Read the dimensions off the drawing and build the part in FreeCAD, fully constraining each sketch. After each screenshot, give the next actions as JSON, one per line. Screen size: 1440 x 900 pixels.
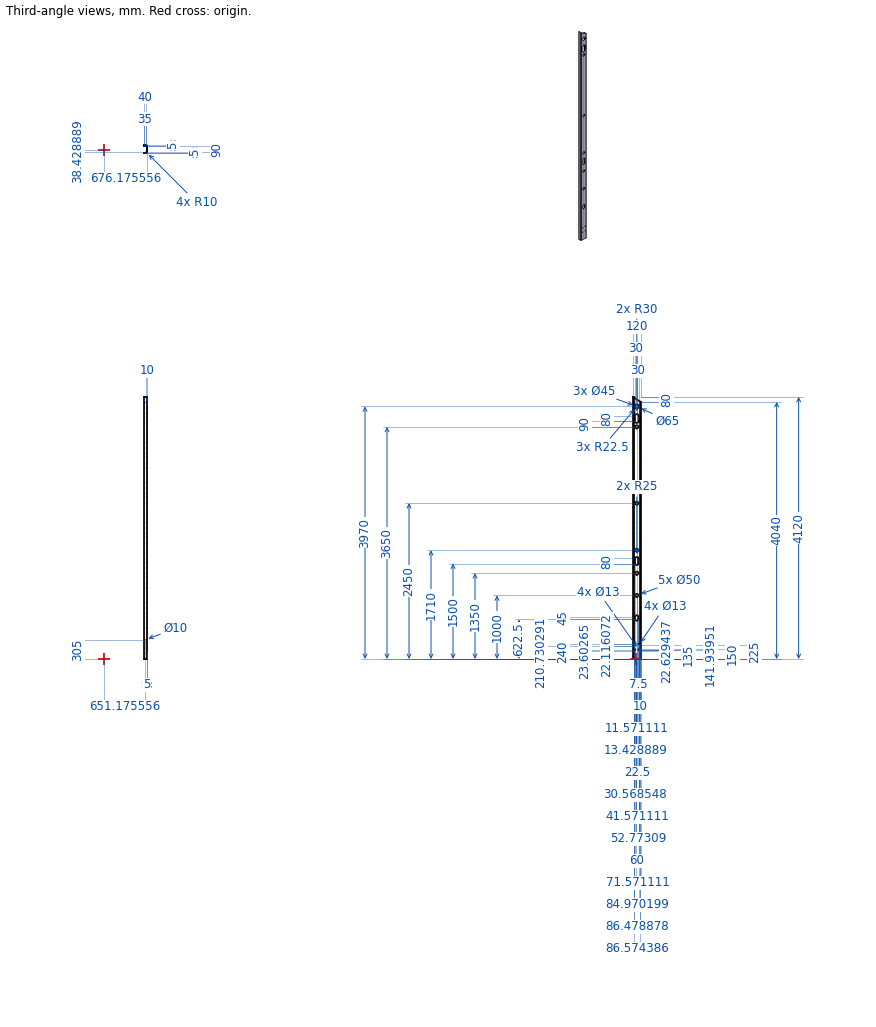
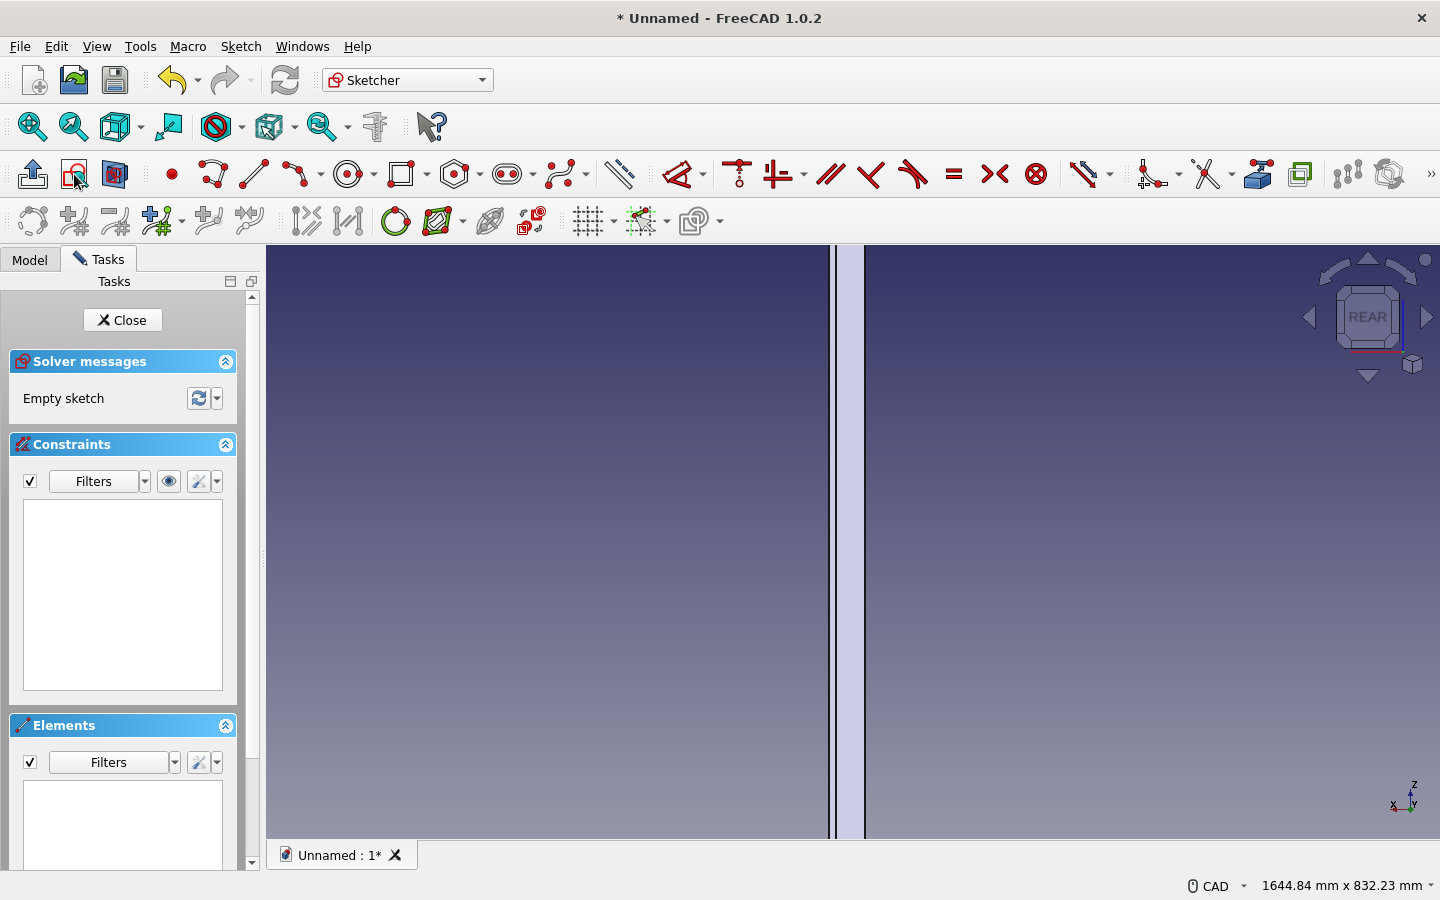
{"action": "scroll", "coordinate": [784, 542], "scroll_direction": "down", "scroll_amount": 5}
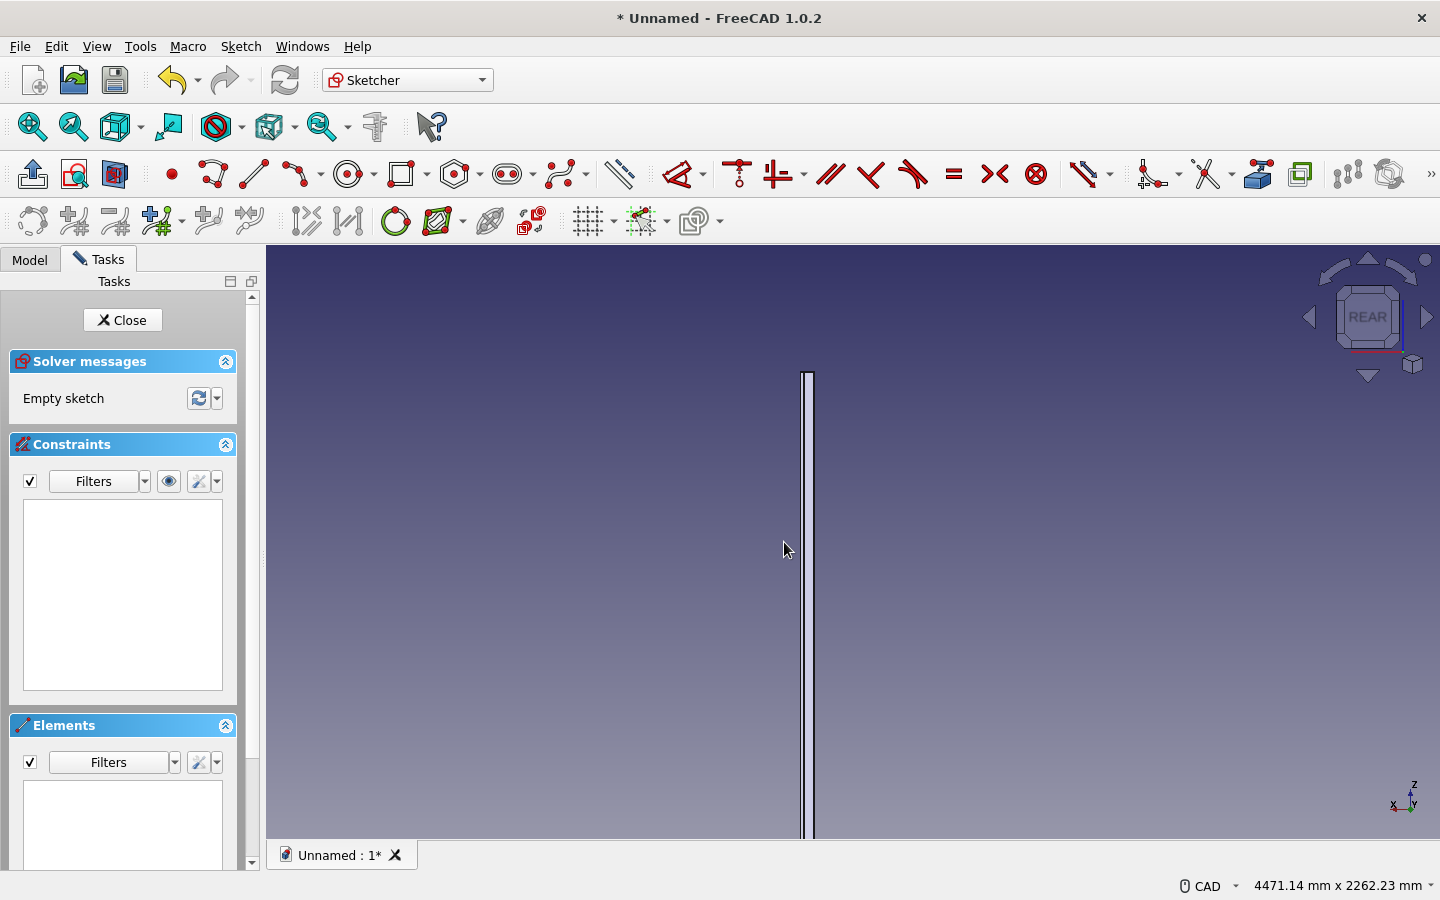
{"action": "scroll", "coordinate": [784, 542], "scroll_direction": "down", "scroll_amount": 5}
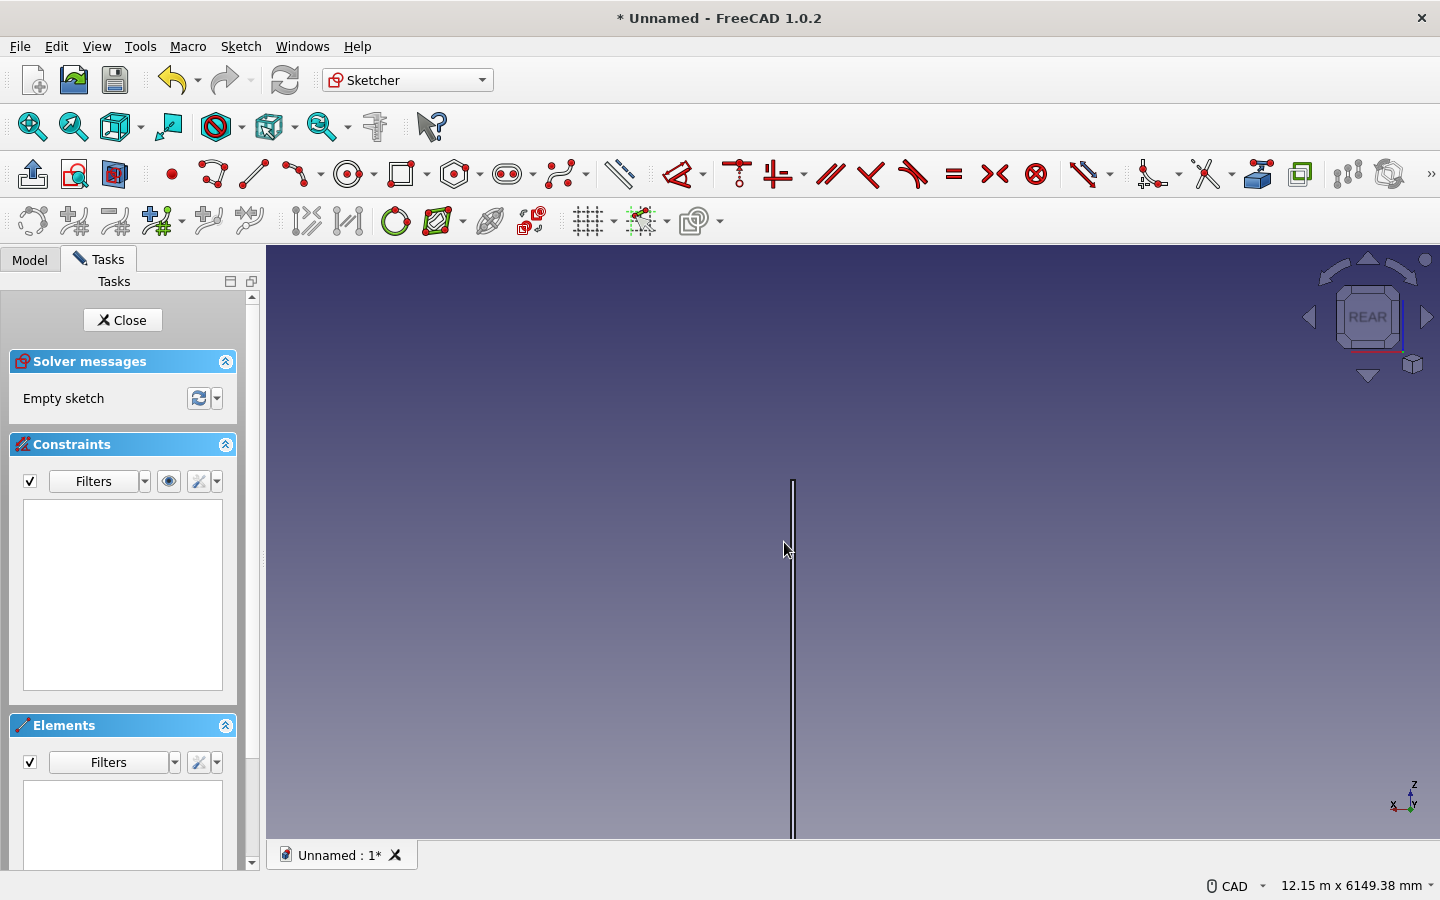
{"action": "scroll", "coordinate": [784, 542], "scroll_direction": "down", "scroll_amount": 5}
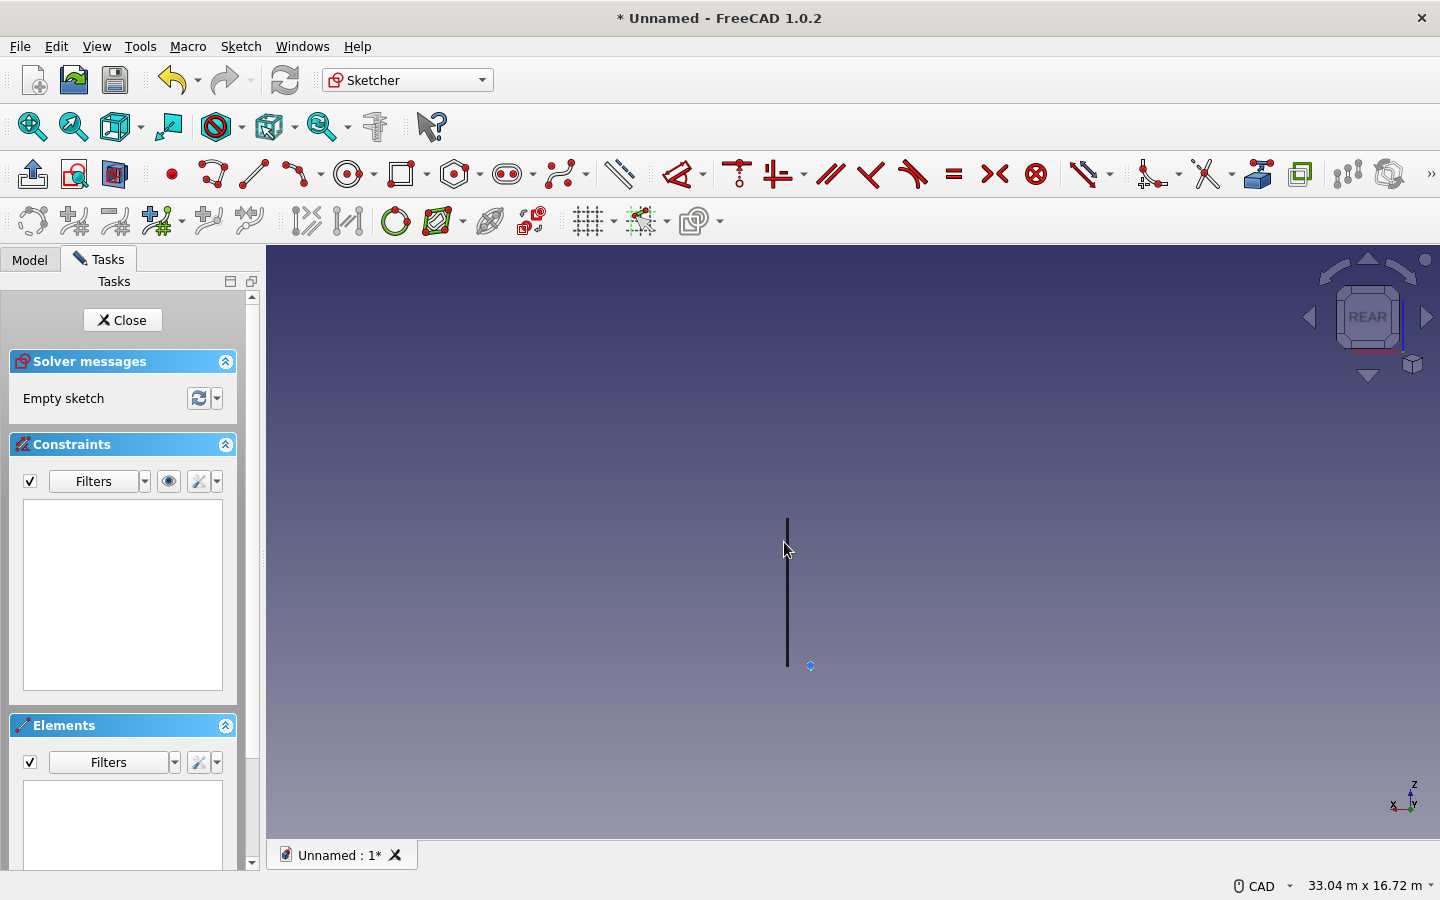
{"action": "scroll", "coordinate": [788, 661], "scroll_direction": "up", "scroll_amount": 15}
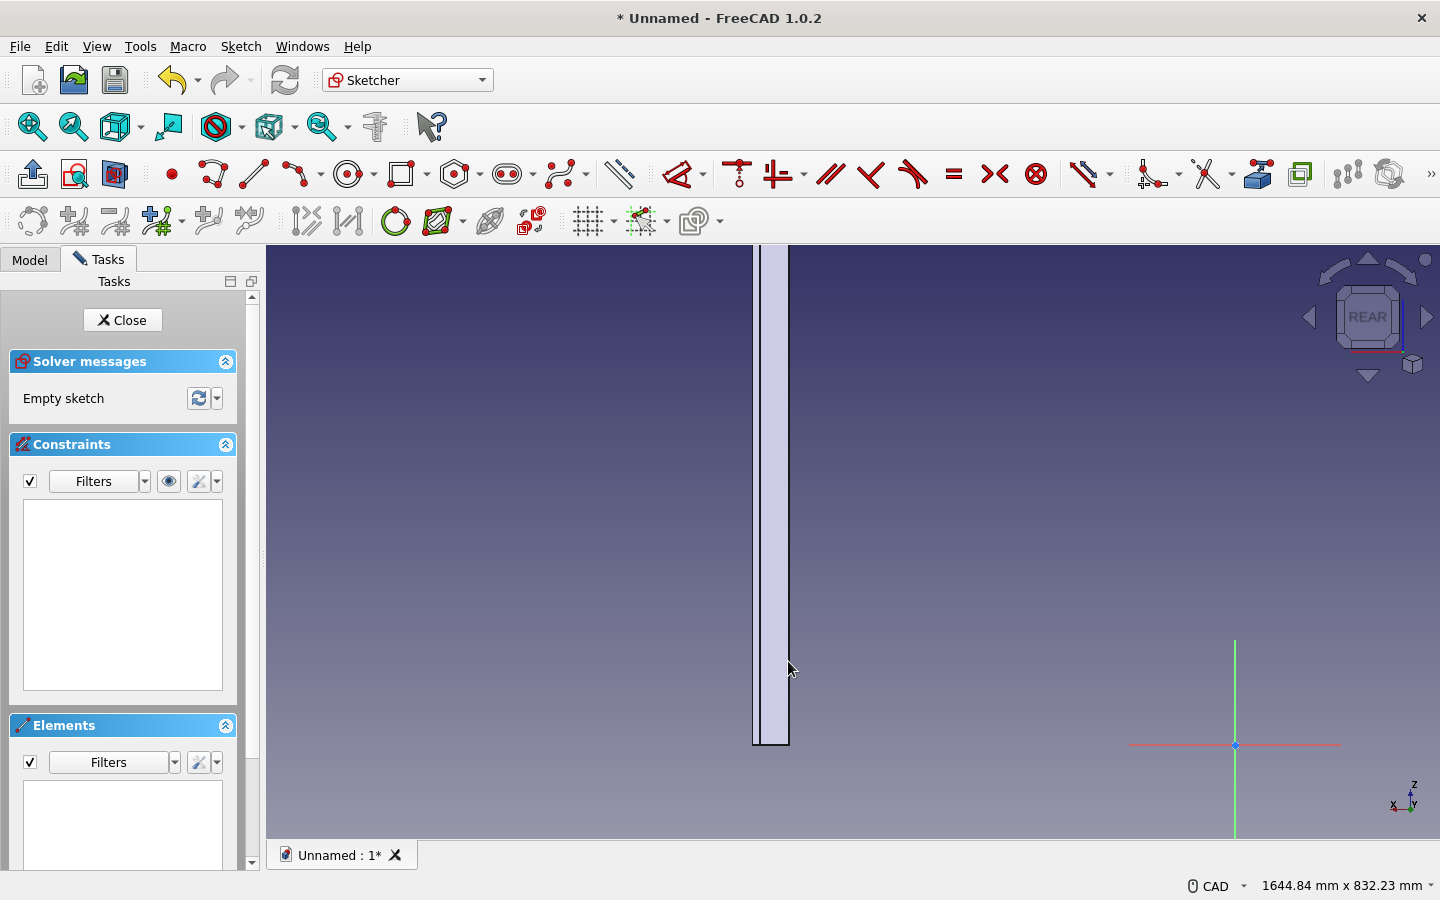
{"action": "scroll", "coordinate": [770, 527], "scroll_direction": "up", "scroll_amount": 15}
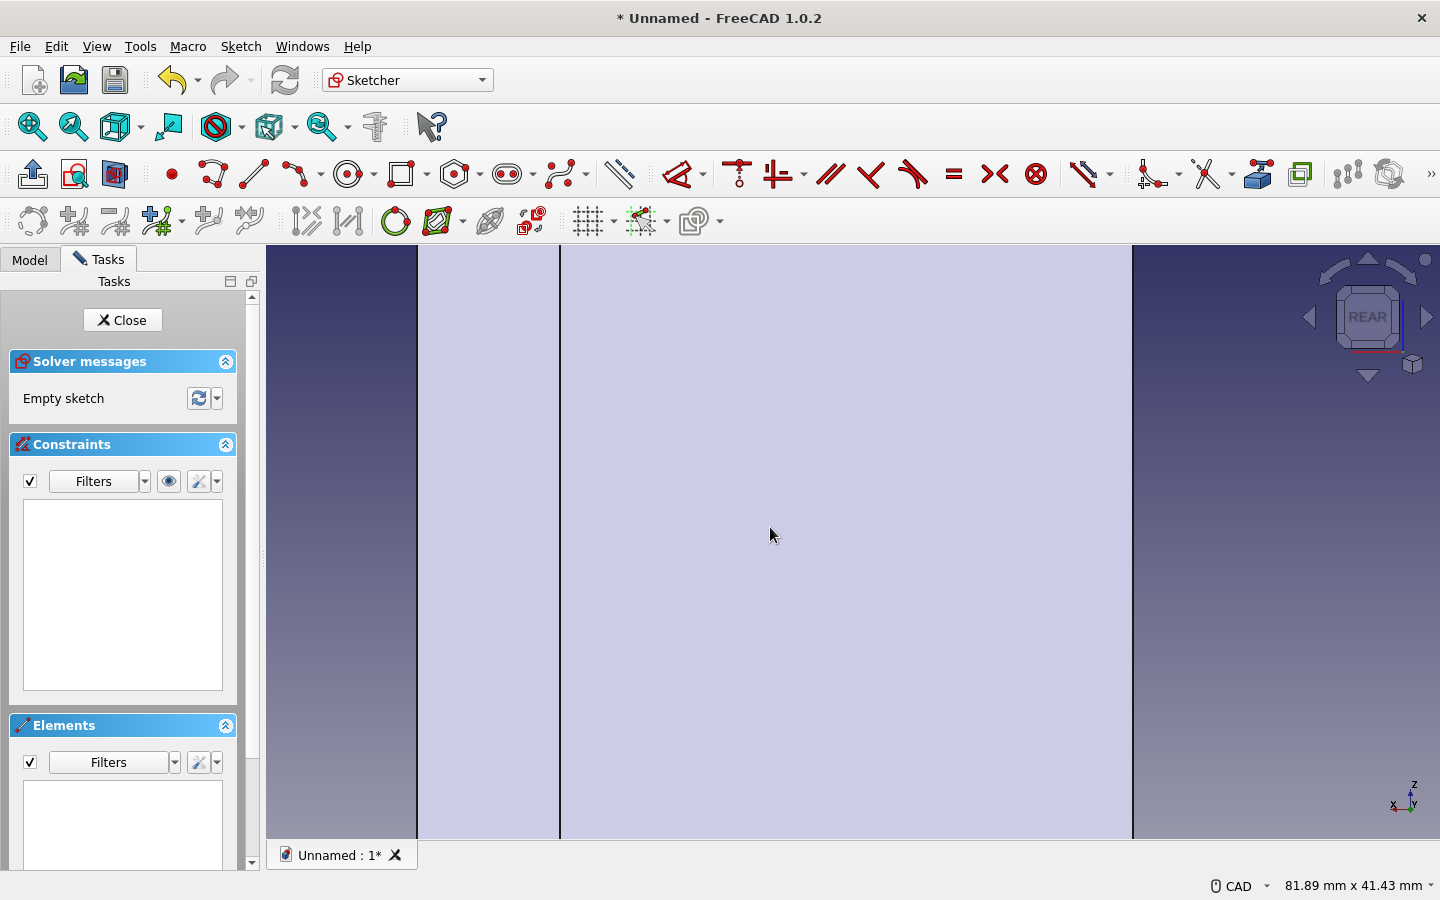
{"action": "left_click", "coordinate": [348, 174]}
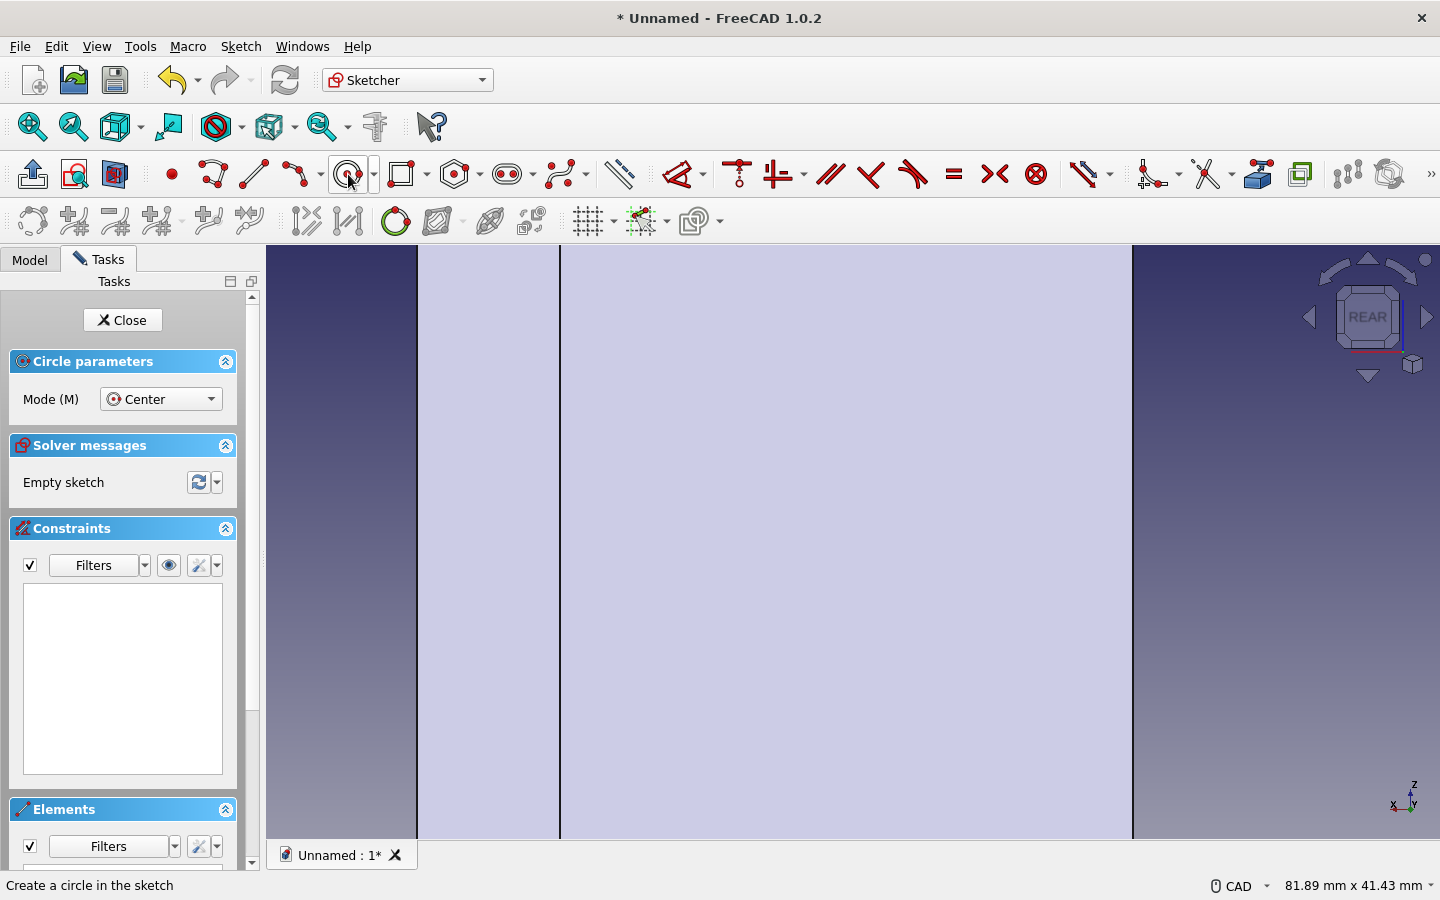
{"action": "left_click", "coordinate": [775, 525]}
{"action": "mouse_move", "coordinate": [826, 474]}